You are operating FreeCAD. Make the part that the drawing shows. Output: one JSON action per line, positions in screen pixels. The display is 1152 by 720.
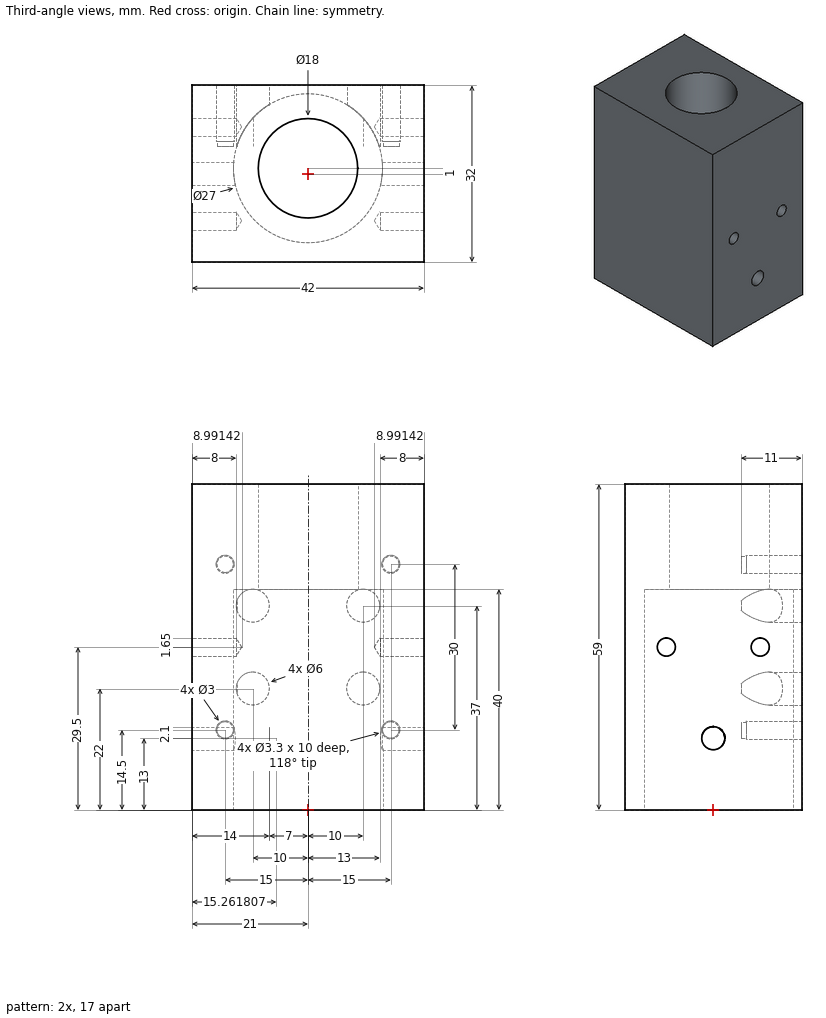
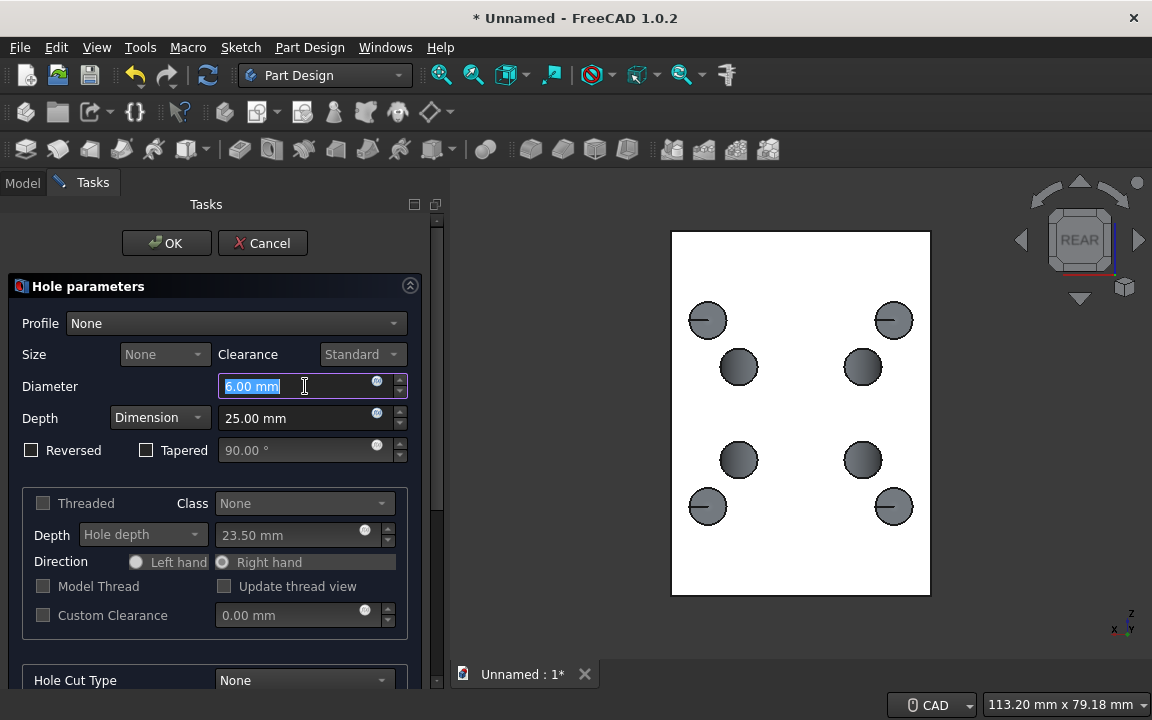
{"action": "type", "text": "3.3"}
{"action": "key", "text": "Tab"}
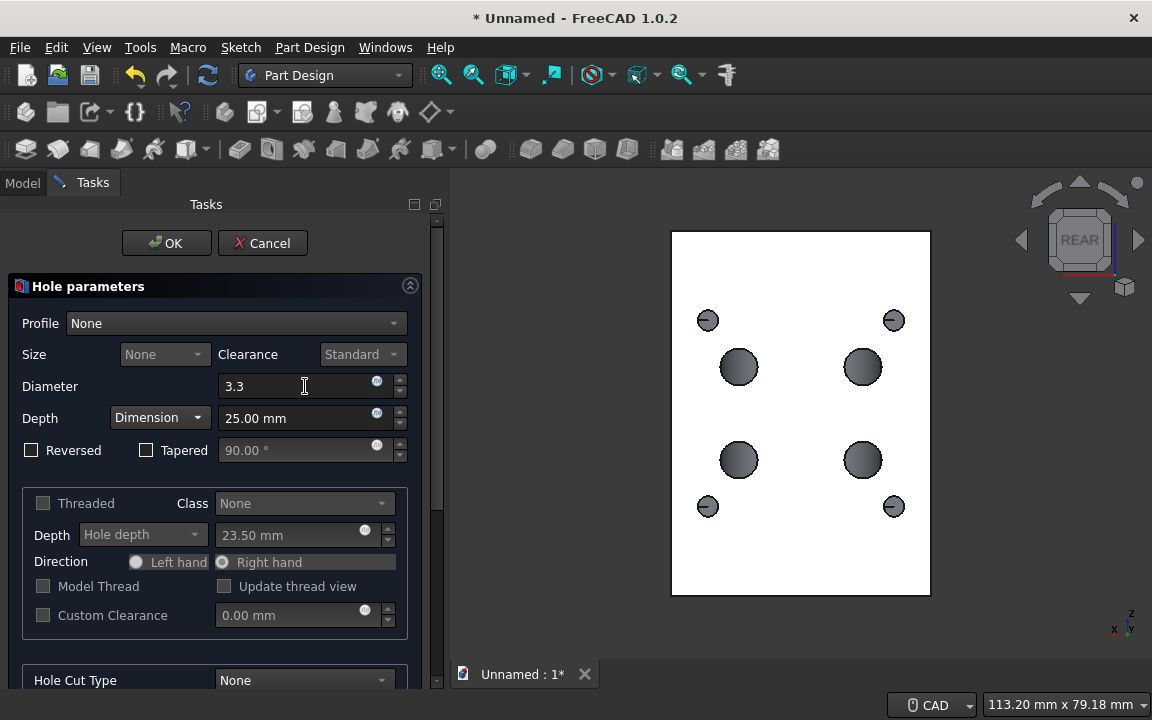
{"action": "triple_click", "coordinate": [305, 418]}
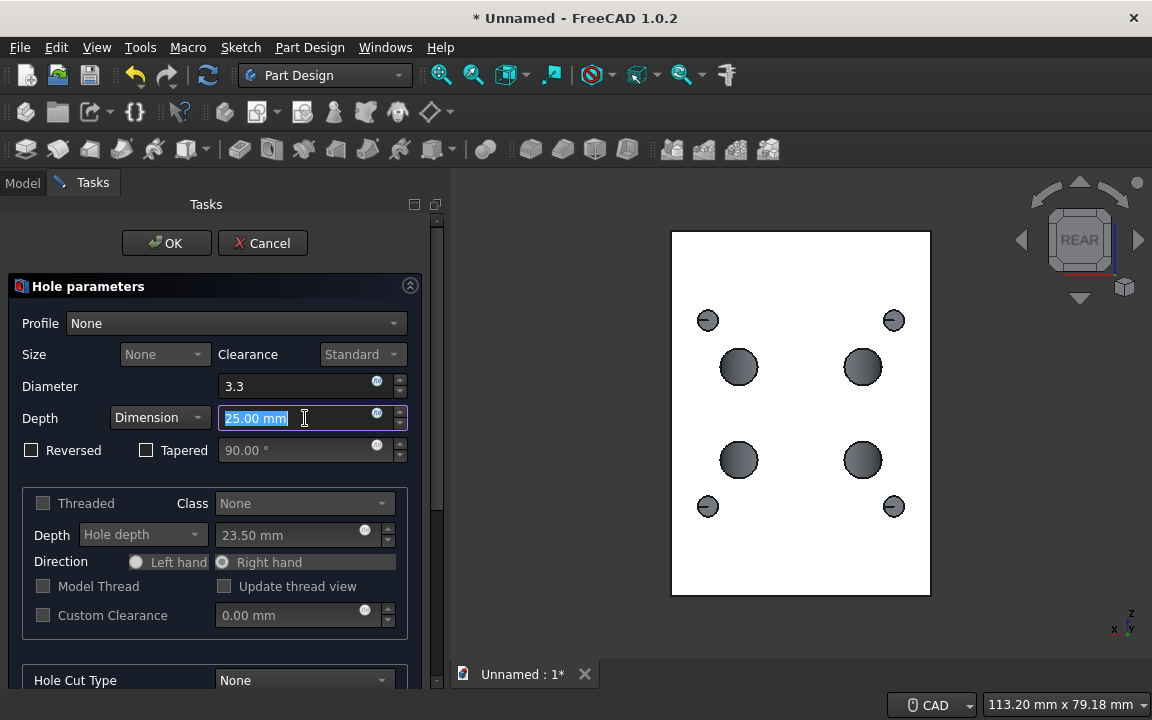
{"action": "type", "text": "10"}
{"action": "key", "text": "Tab"}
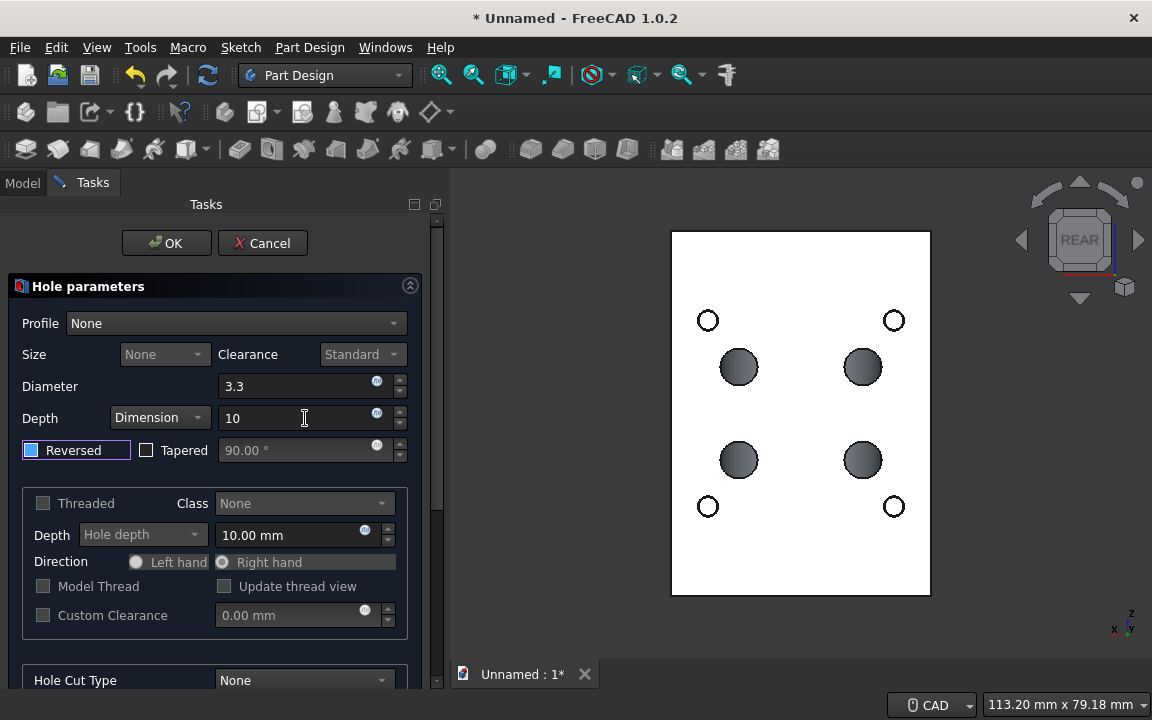
{"action": "left_click", "coordinate": [167, 243]}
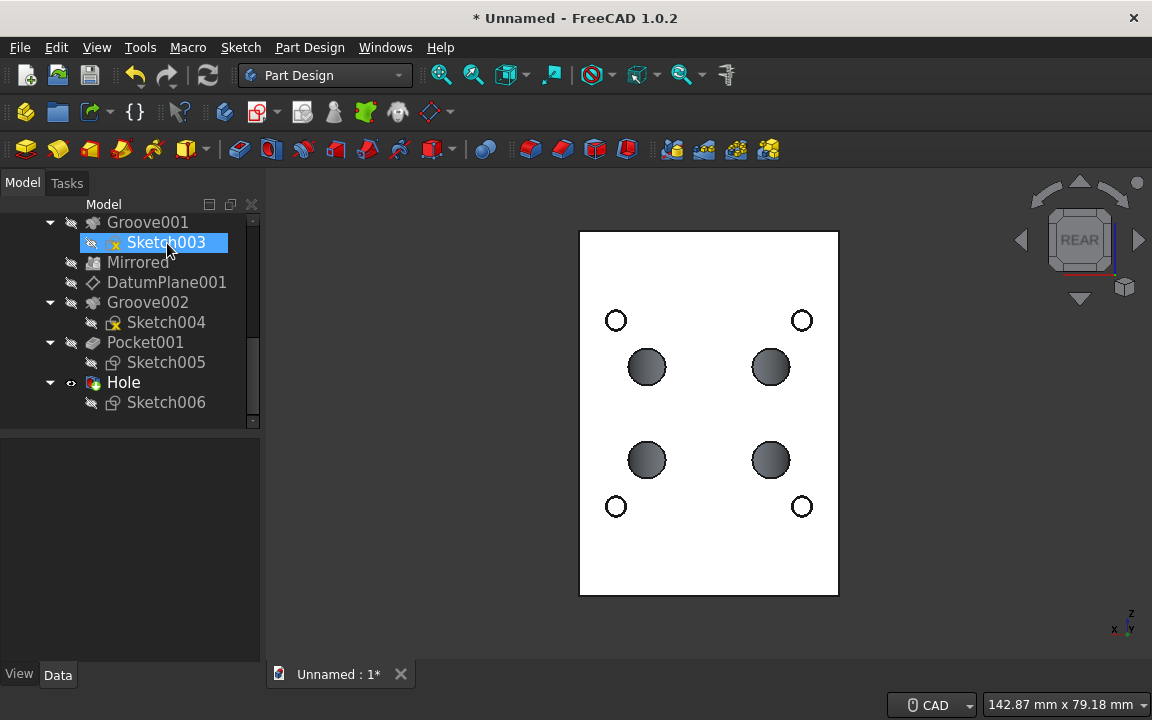
{"action": "key", "text": "0"}